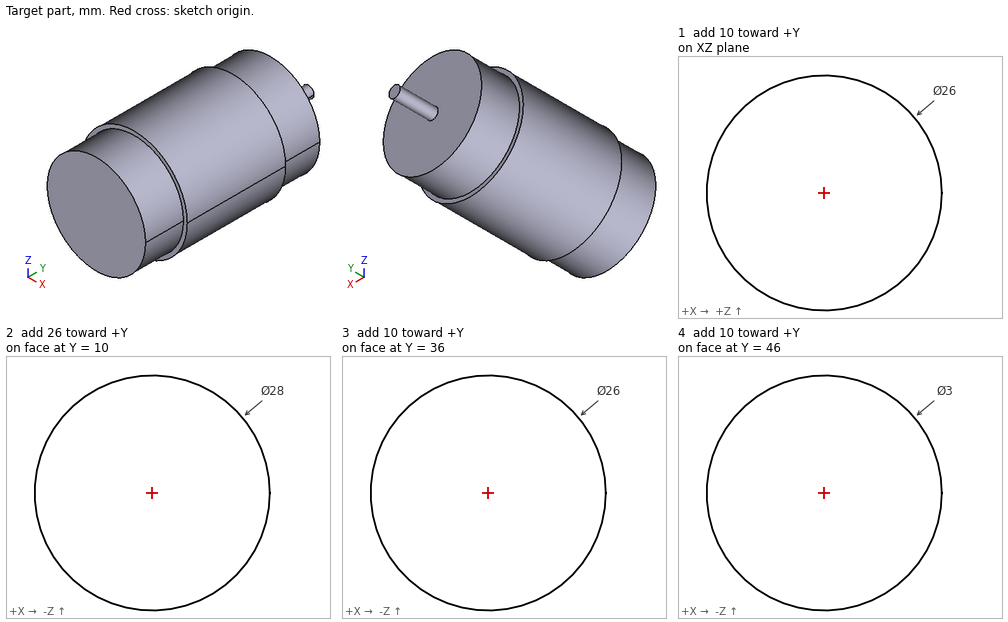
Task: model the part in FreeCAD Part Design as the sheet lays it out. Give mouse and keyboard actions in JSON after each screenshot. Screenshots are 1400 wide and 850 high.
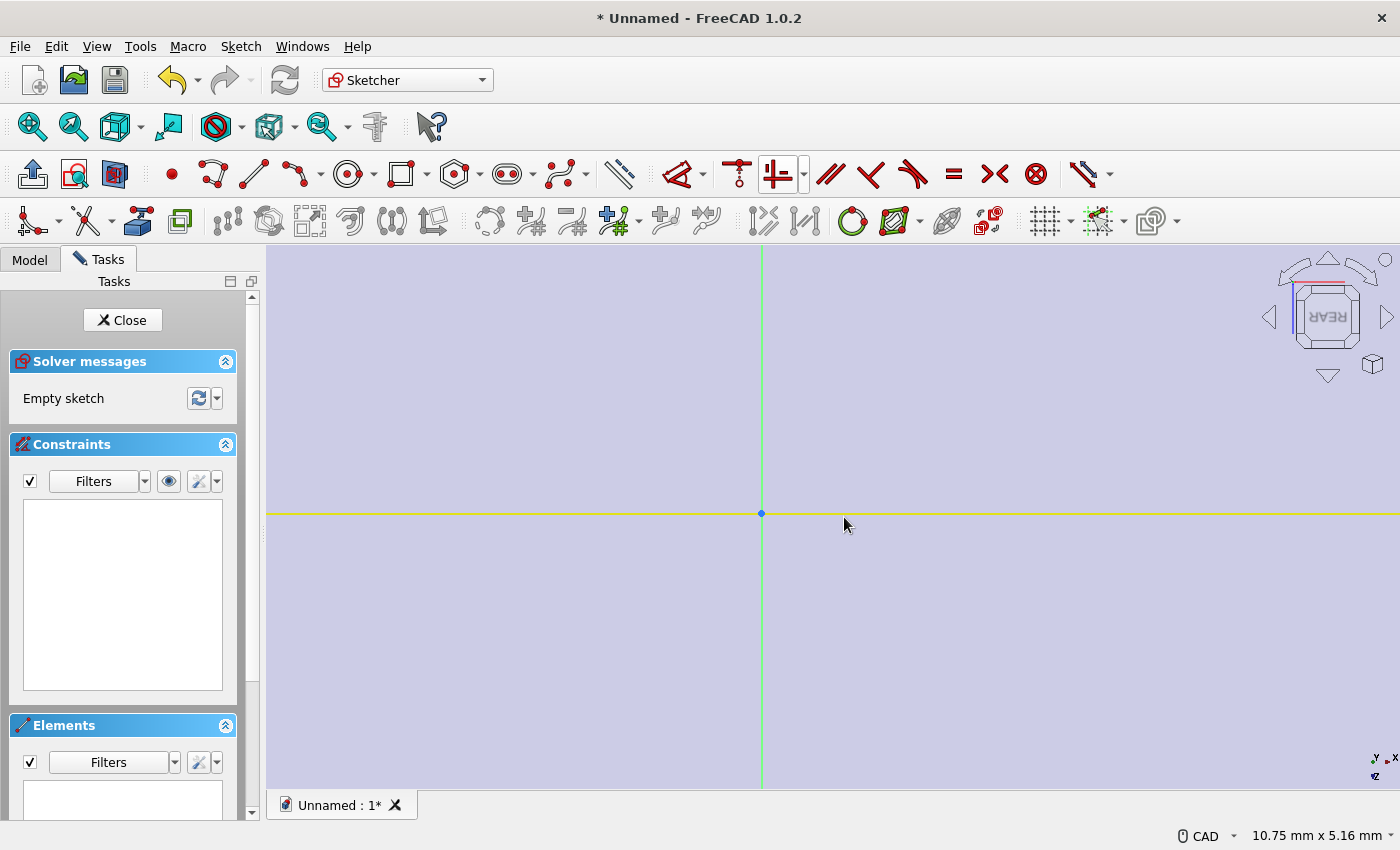
{"action": "left_click", "coordinate": [348, 174]}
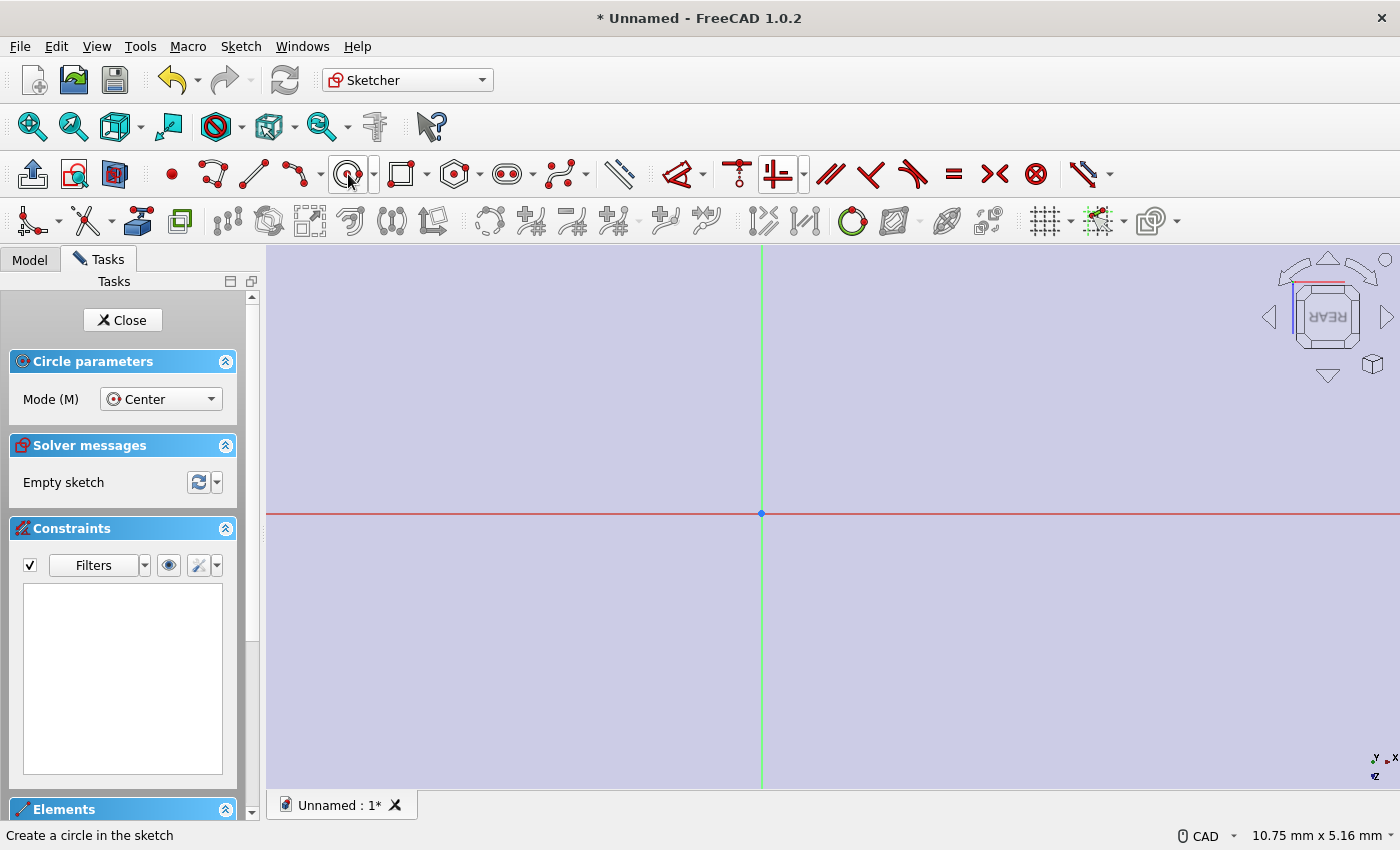
{"action": "left_click", "coordinate": [762, 514]}
{"action": "mouse_move", "coordinate": [874, 402]}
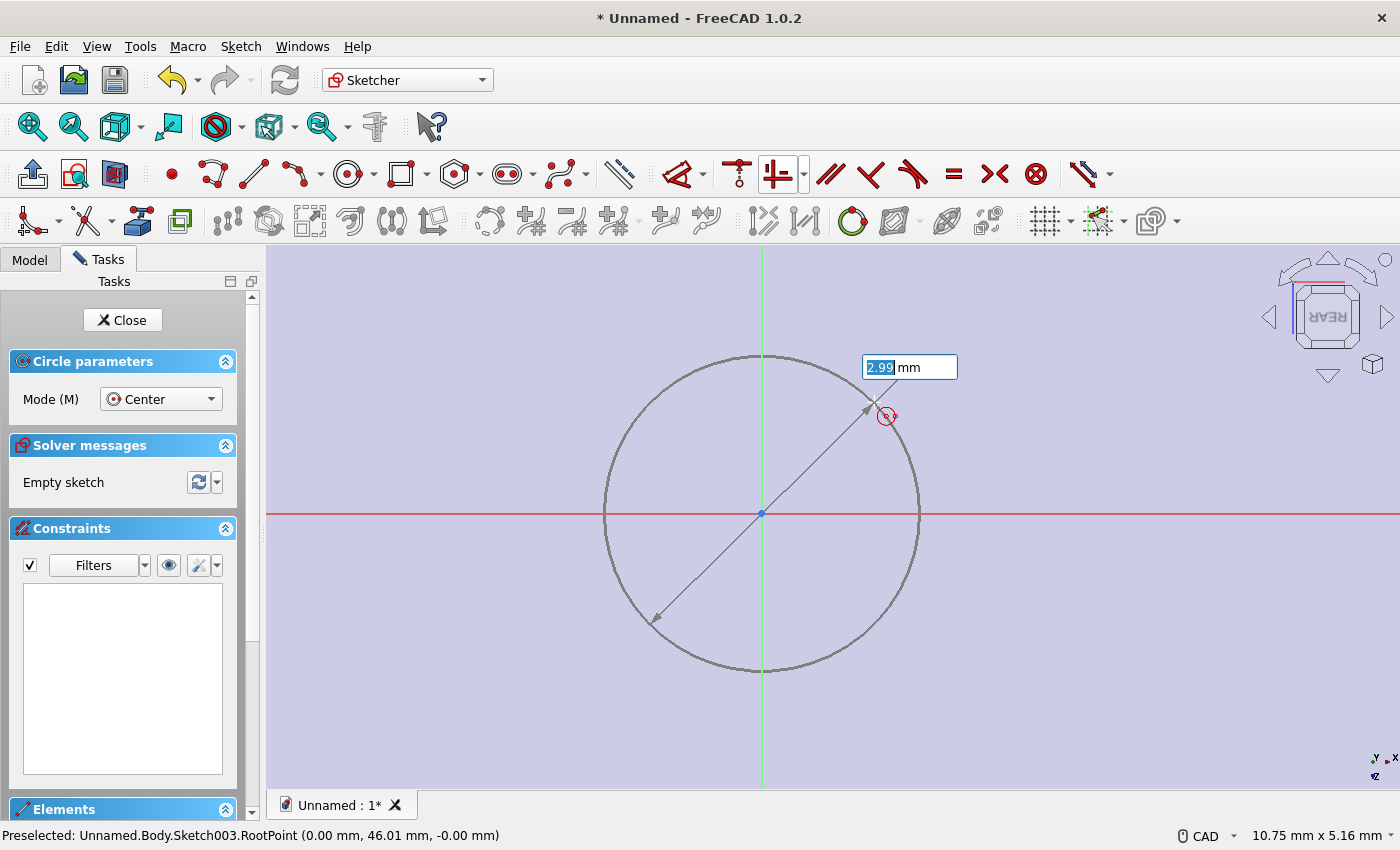
{"action": "type", "text": "3"}
{"action": "key", "text": "Return"}
{"action": "key", "text": "Escape"}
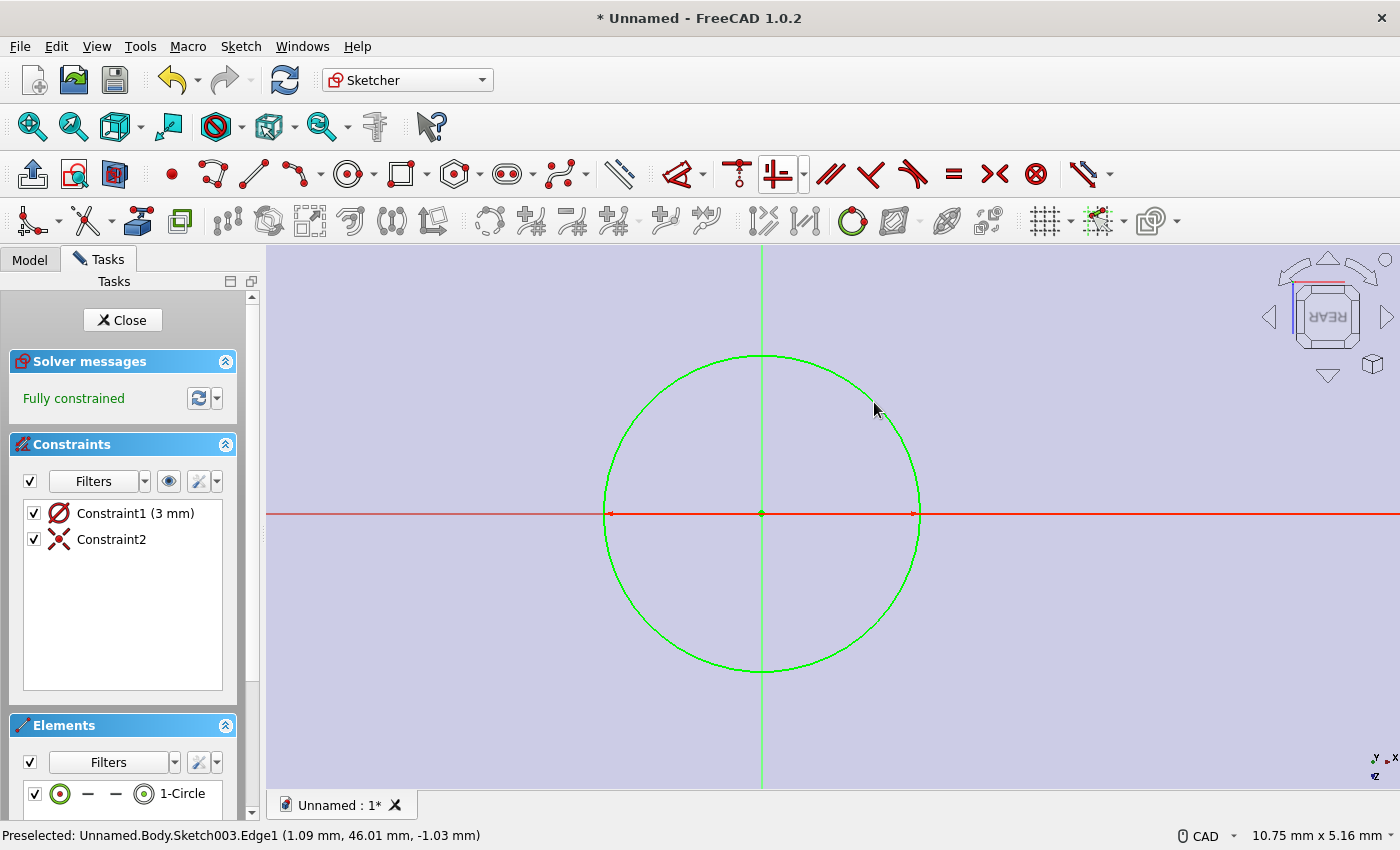
{"action": "left_click", "coordinate": [123, 320]}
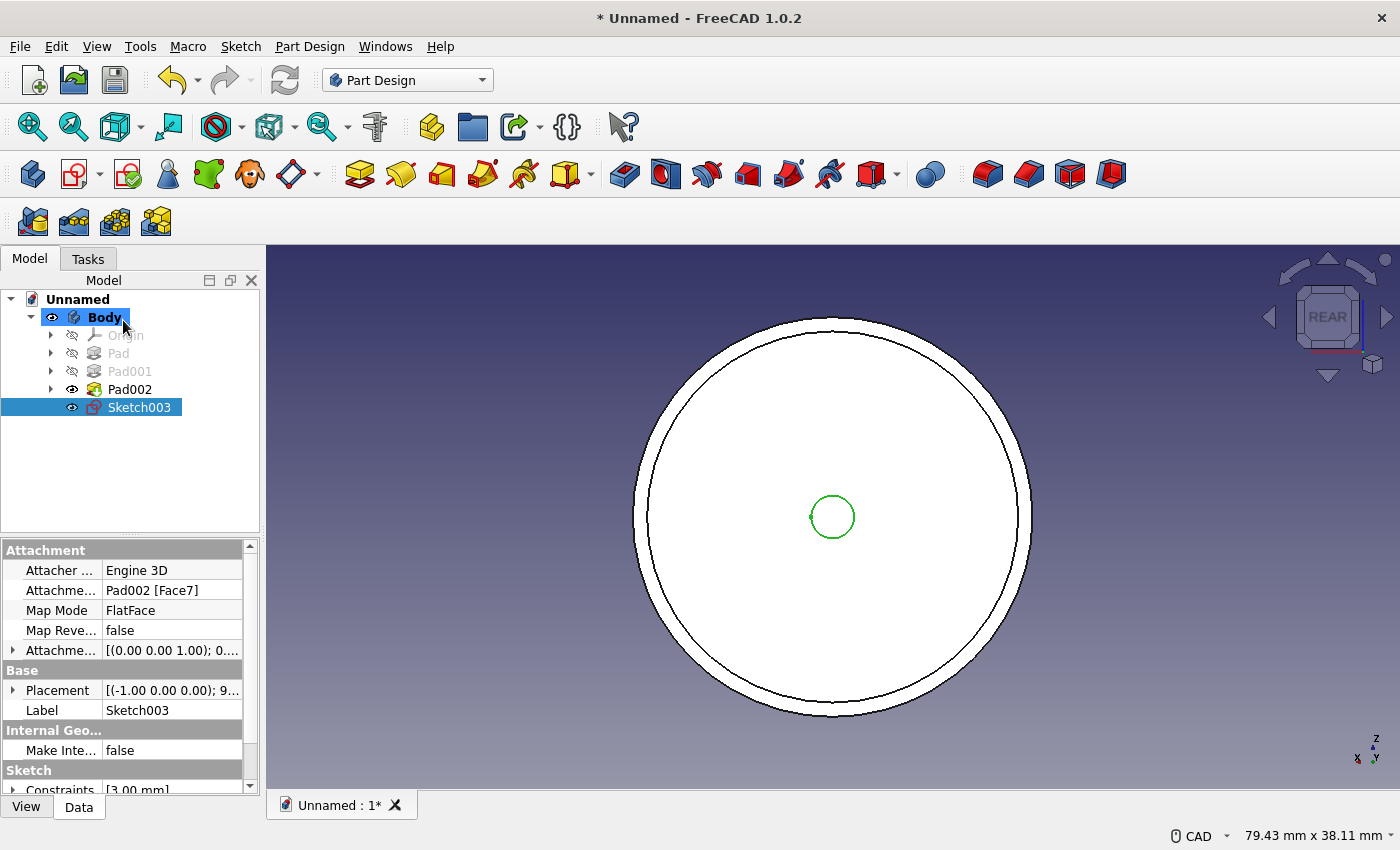
{"action": "left_click", "coordinate": [360, 174]}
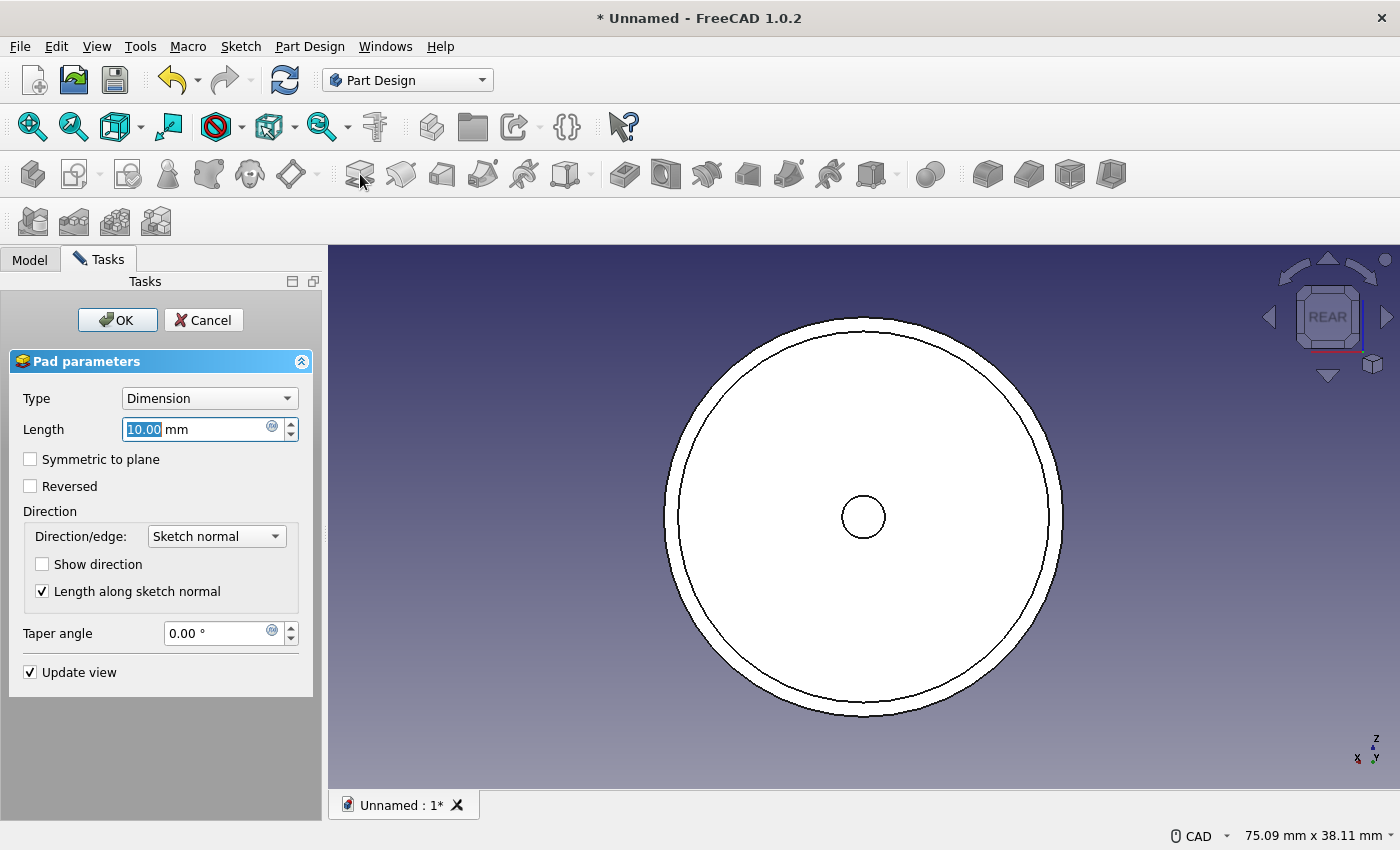
{"action": "type", "text": "10"}
{"action": "key", "text": "Tab"}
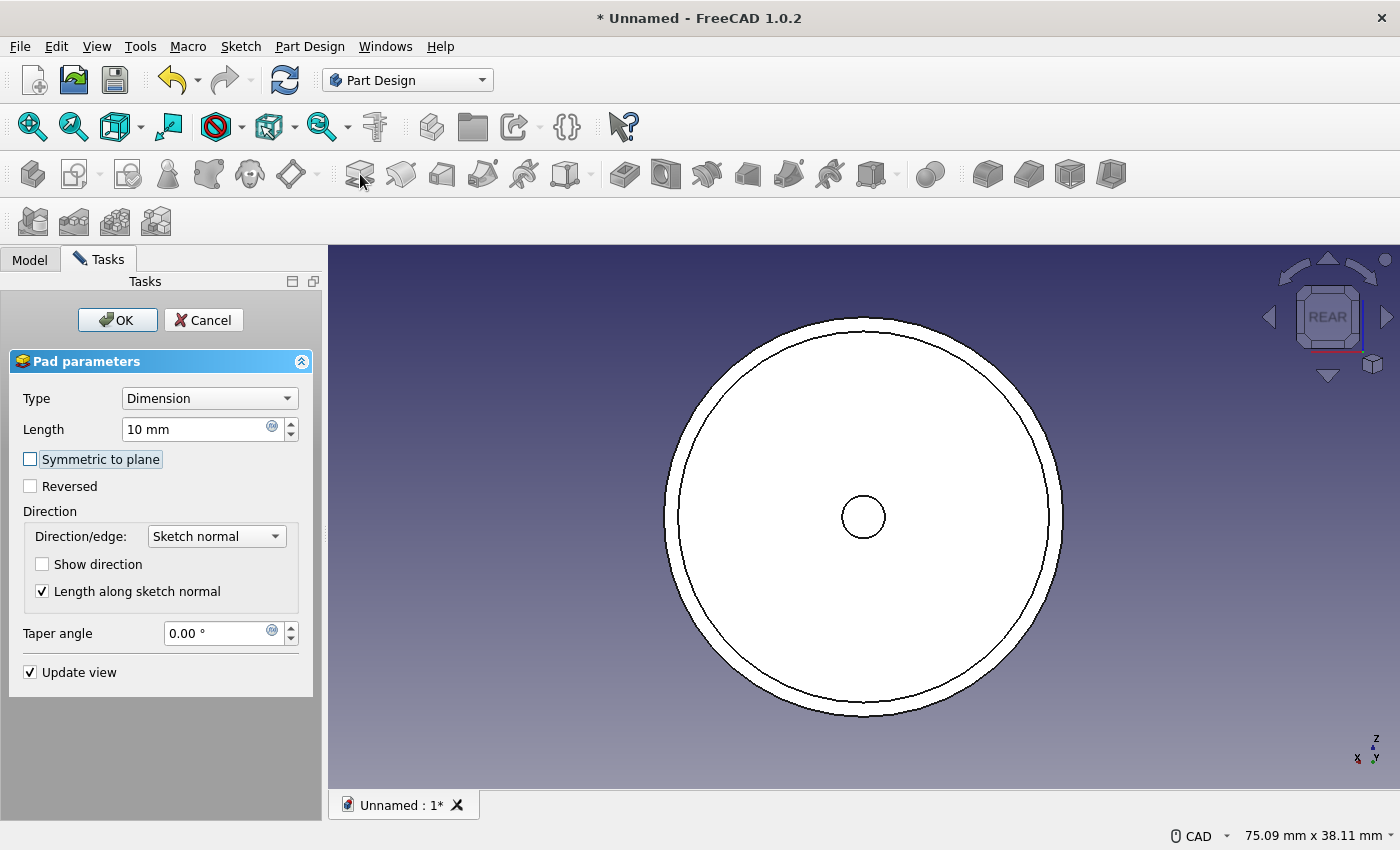
{"action": "left_click", "coordinate": [118, 320]}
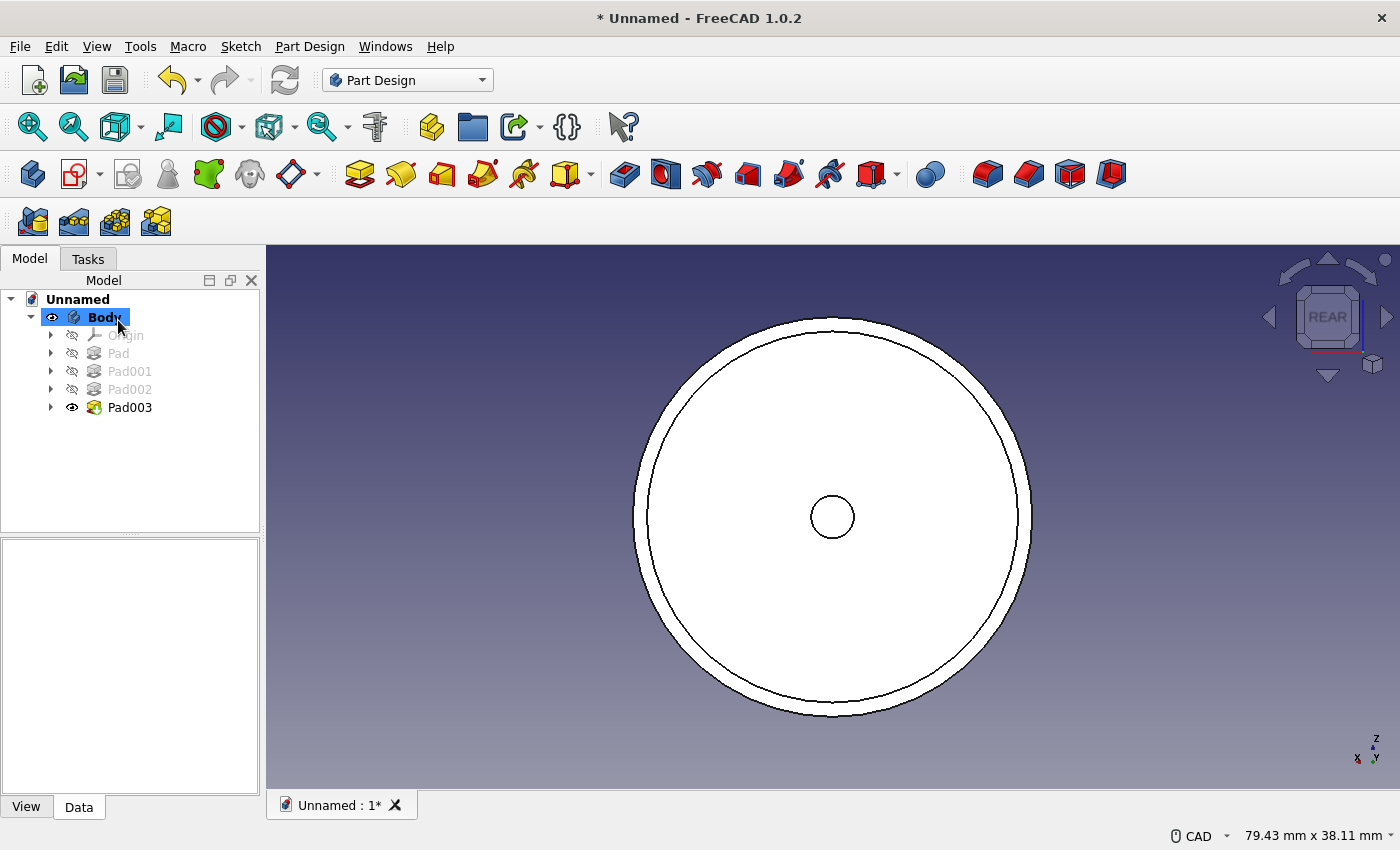
{"action": "key", "text": "0"}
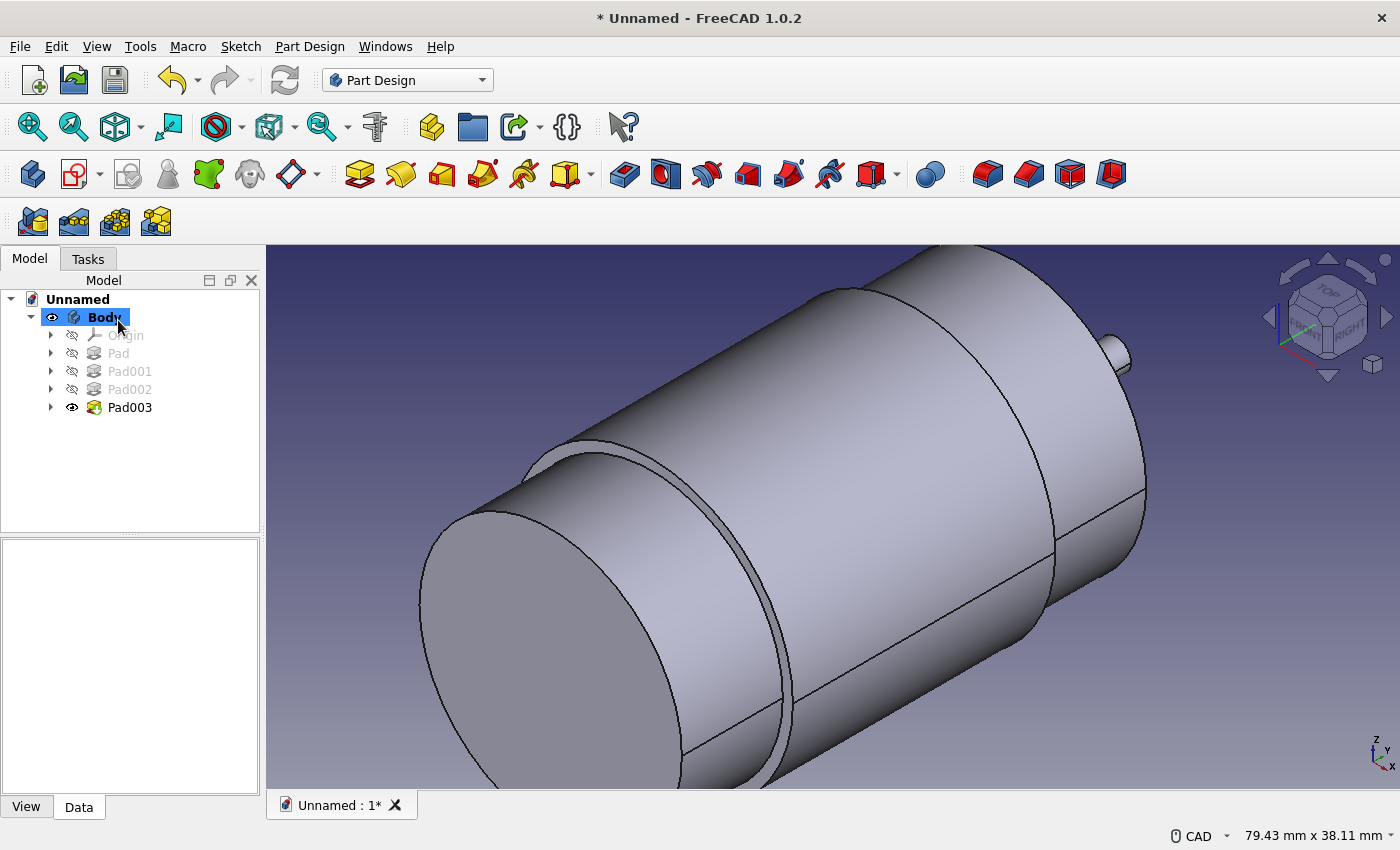
{"action": "left_click", "coordinate": [33, 128]}